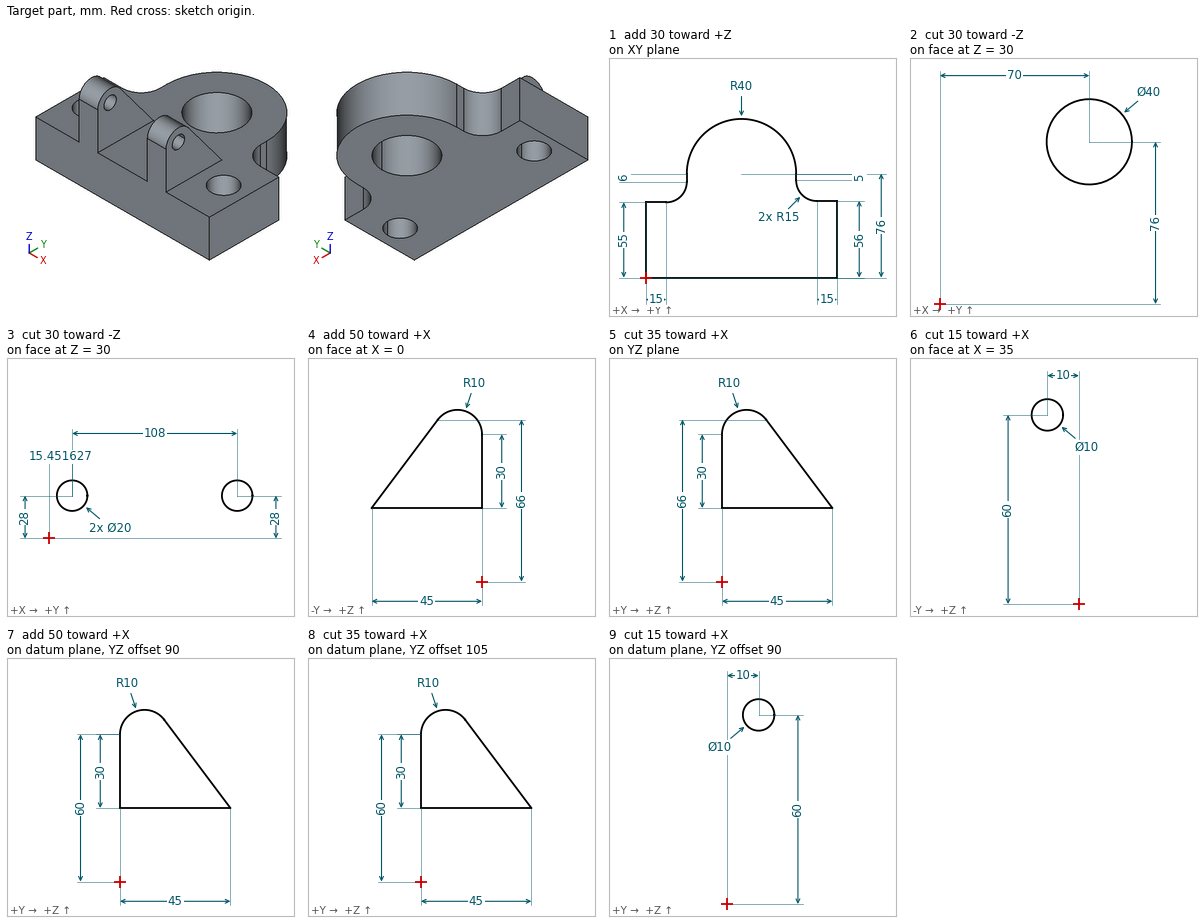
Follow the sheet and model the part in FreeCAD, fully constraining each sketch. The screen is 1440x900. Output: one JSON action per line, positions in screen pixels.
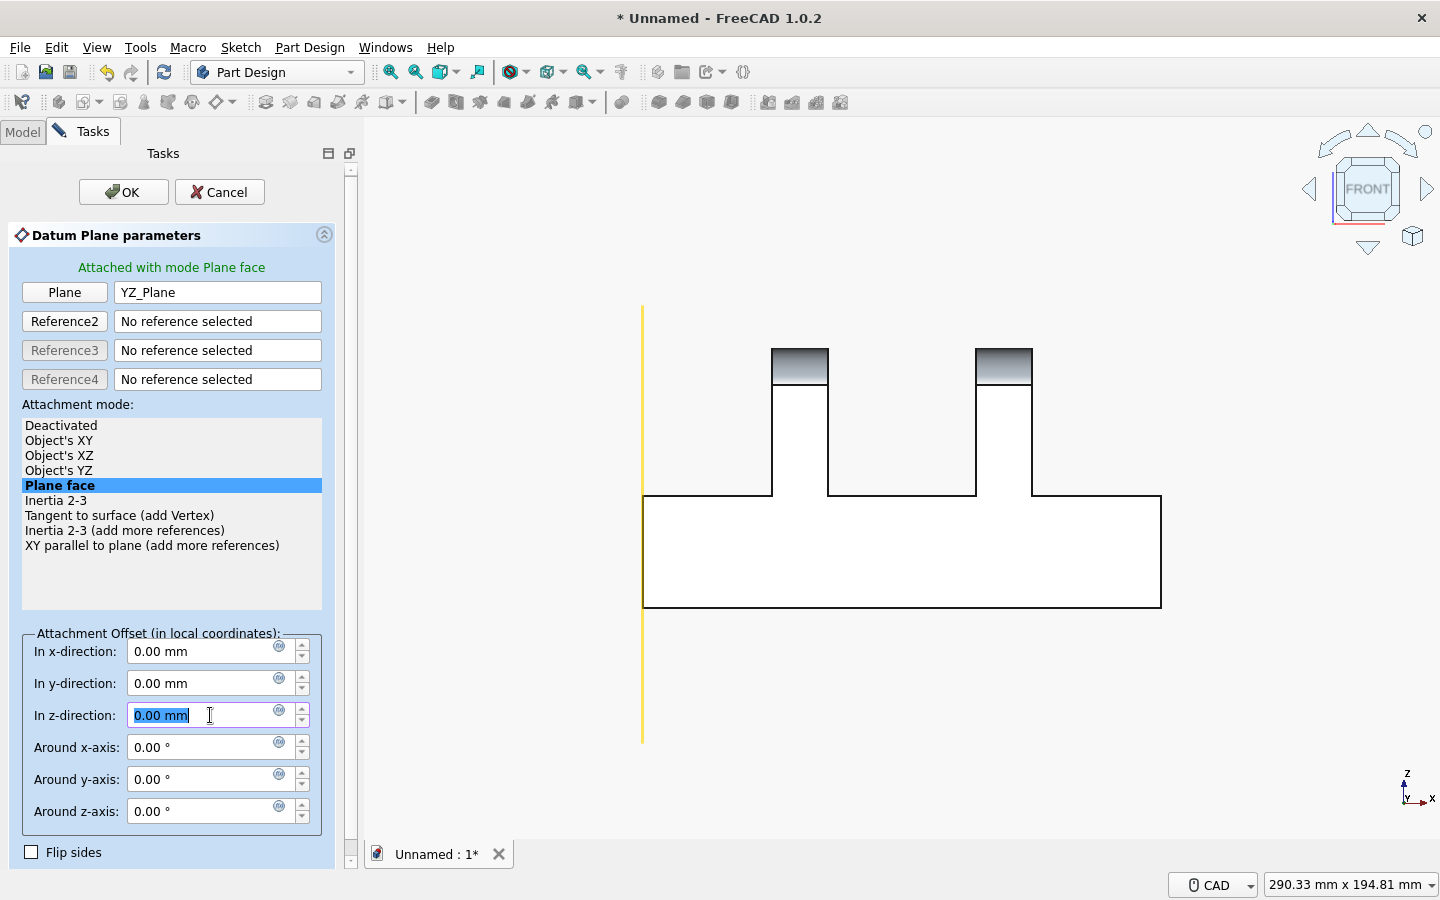
{"action": "type", "text": "90"}
{"action": "key", "text": "Tab"}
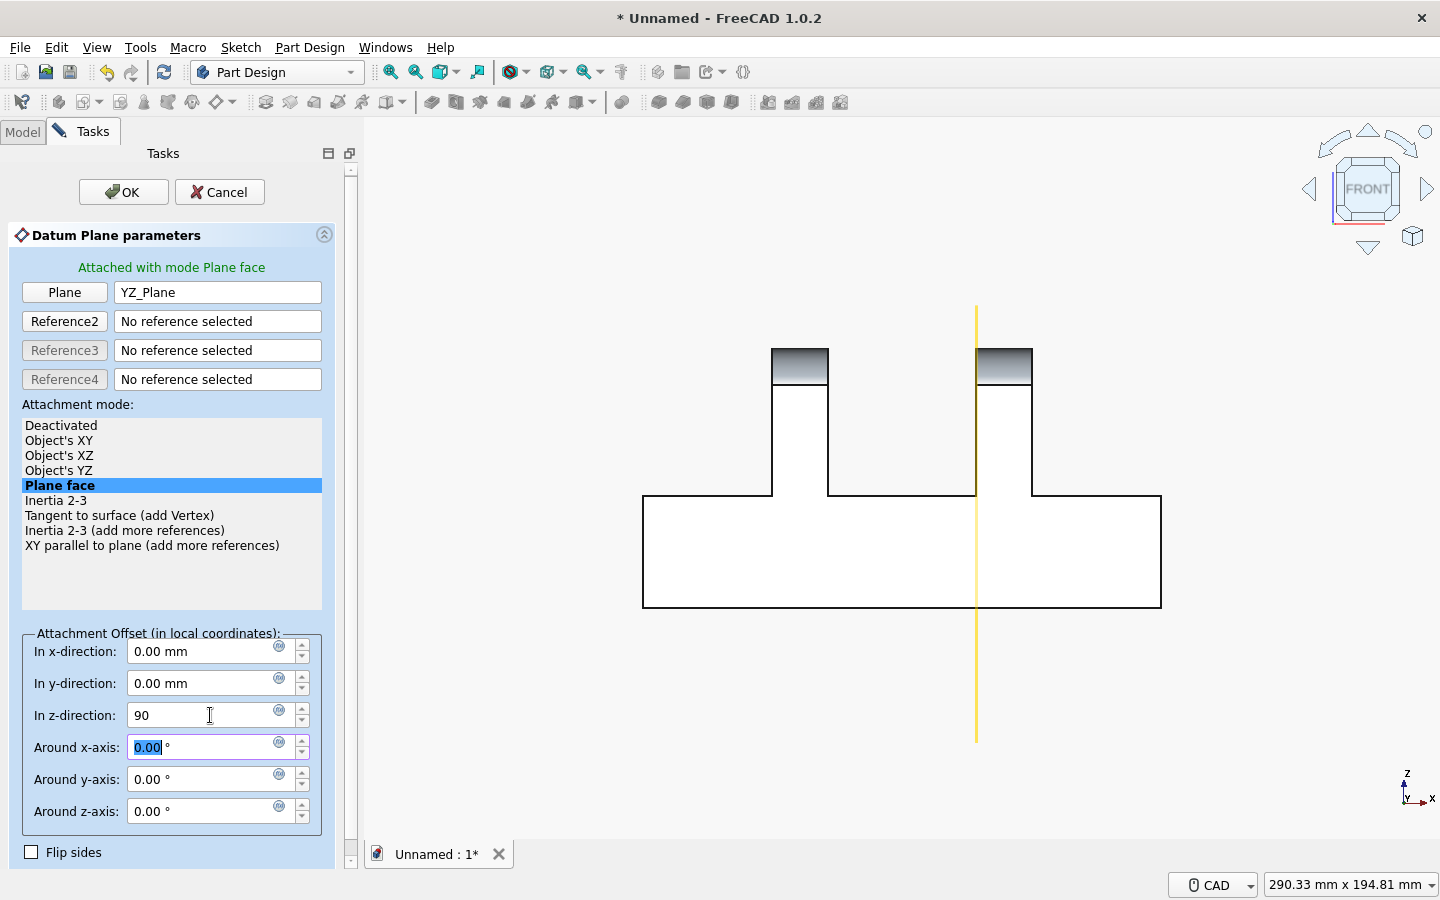
{"action": "left_click", "coordinate": [124, 192]}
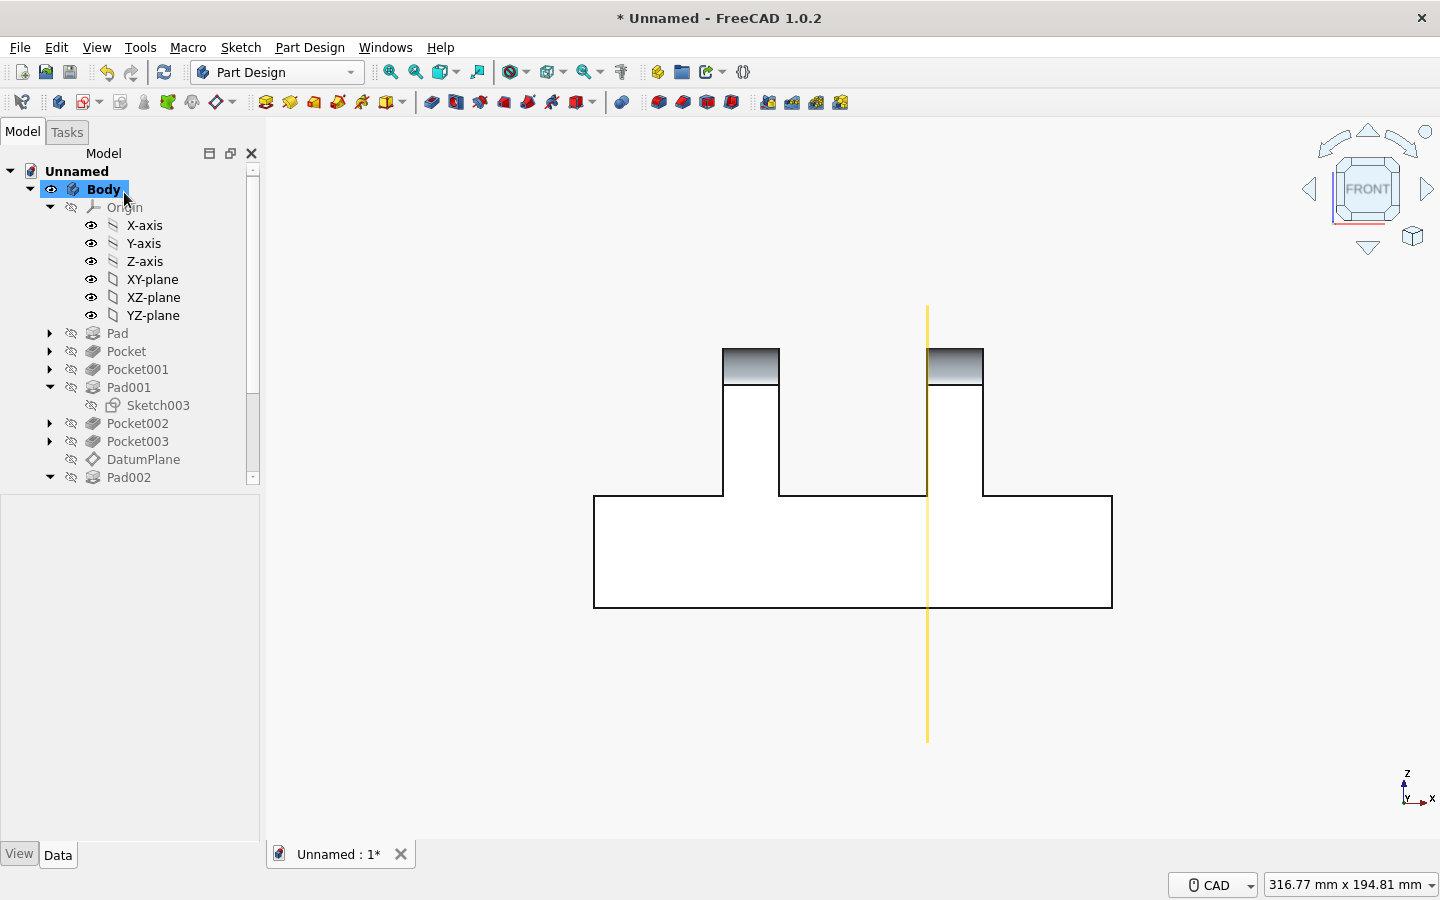
{"action": "scroll", "coordinate": [100, 329], "scroll_direction": "down", "scroll_amount": 3}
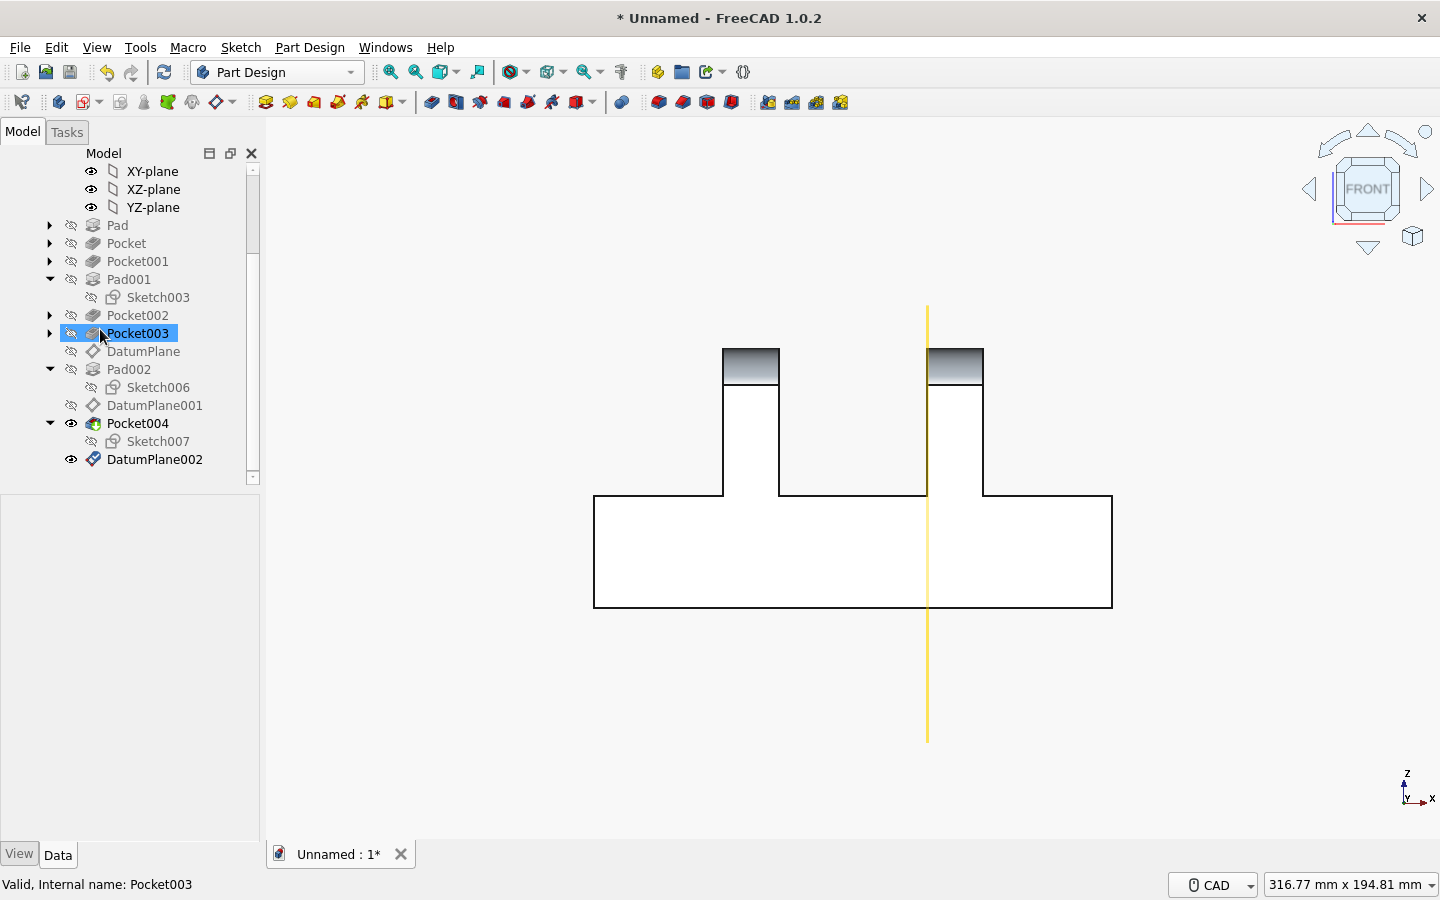
{"action": "left_click", "coordinate": [116, 459]}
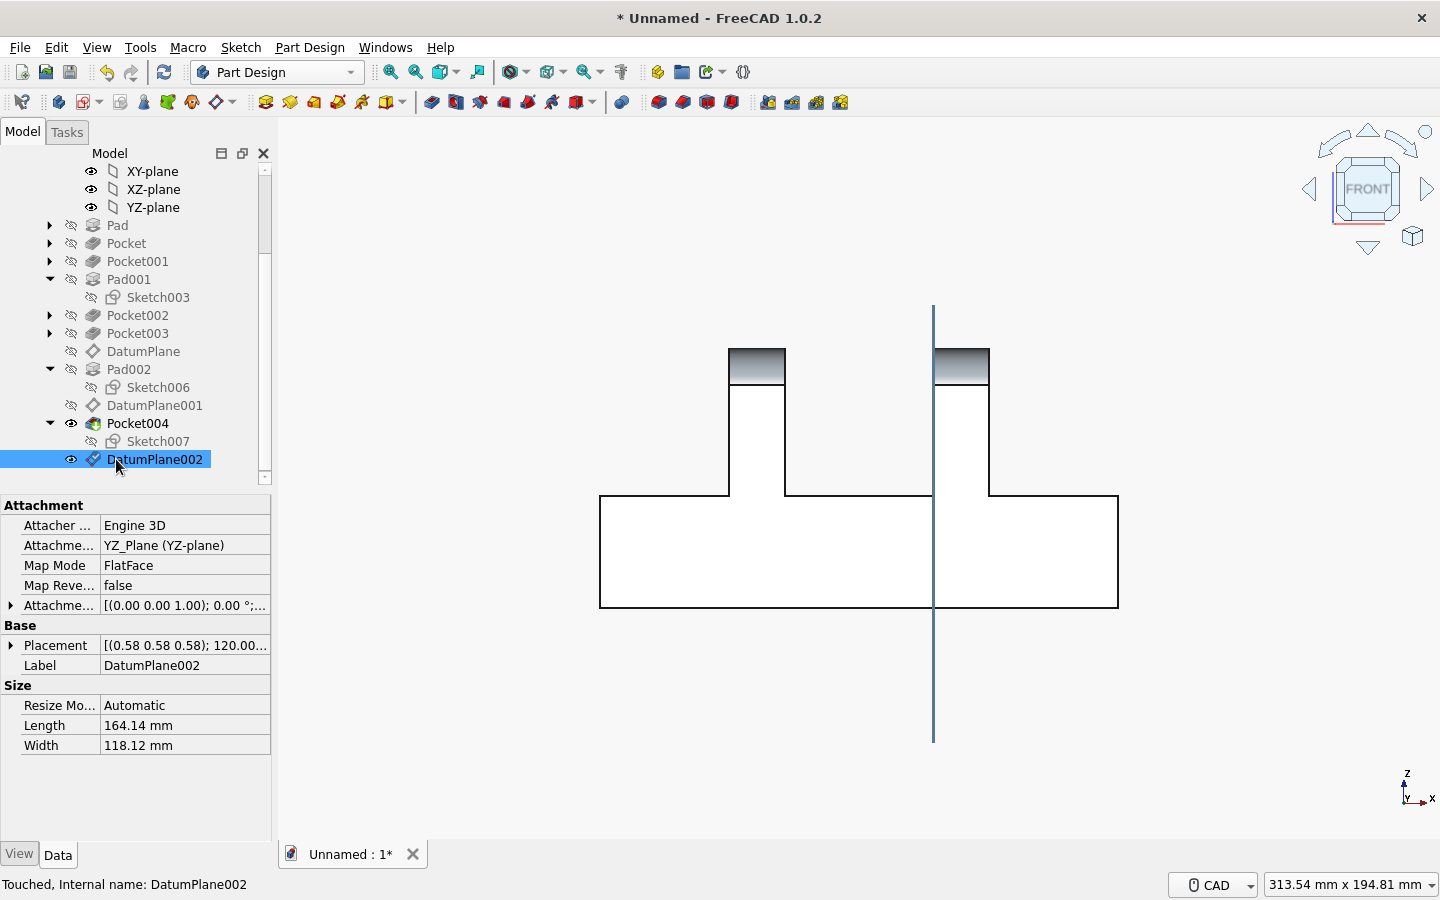
{"action": "left_click", "coordinate": [84, 102]}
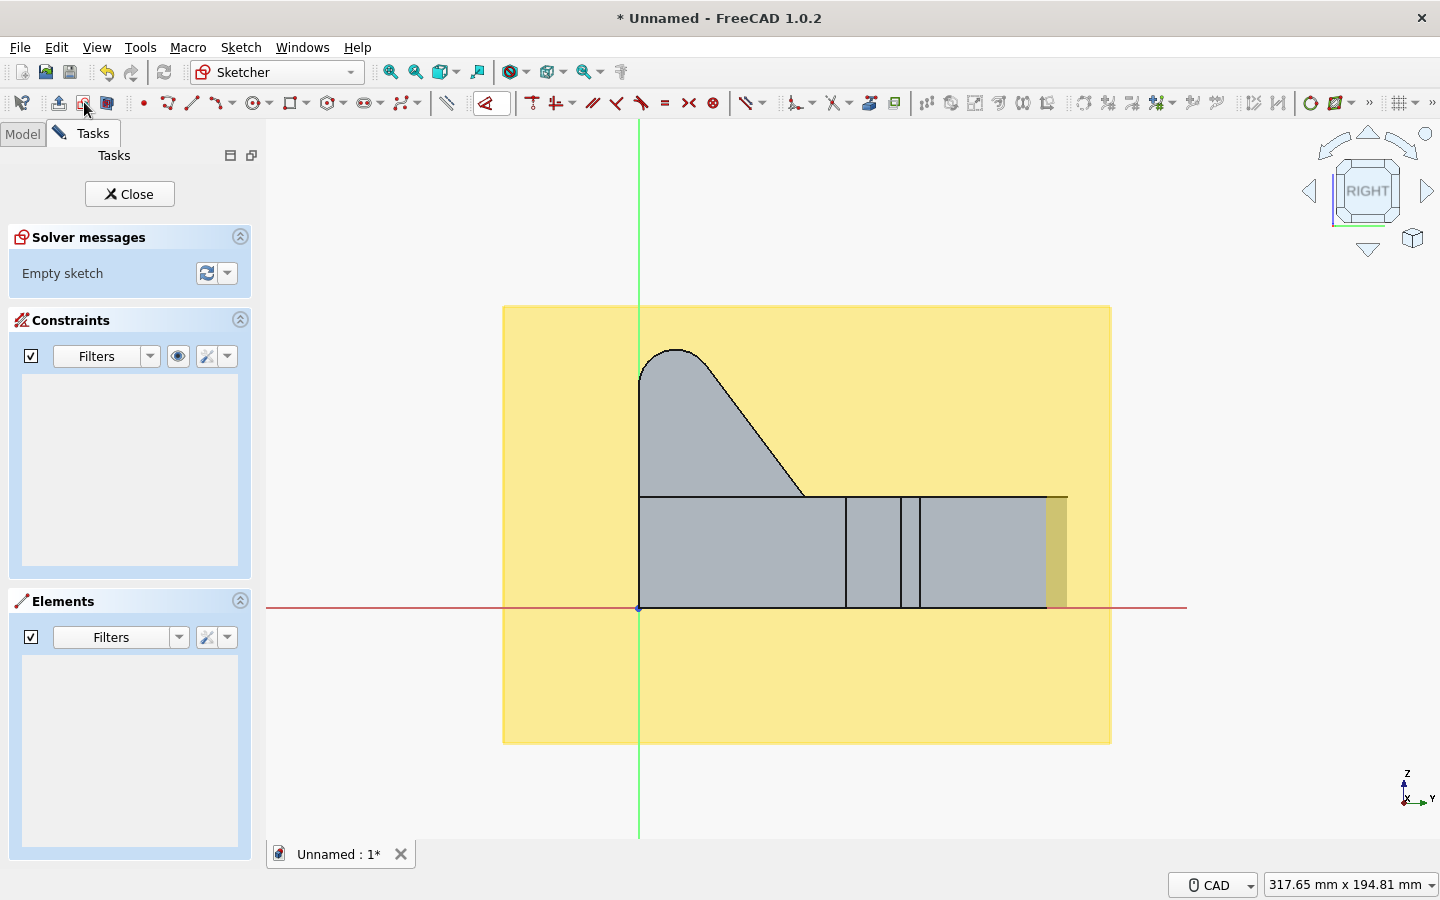
{"action": "key", "text": "q s"}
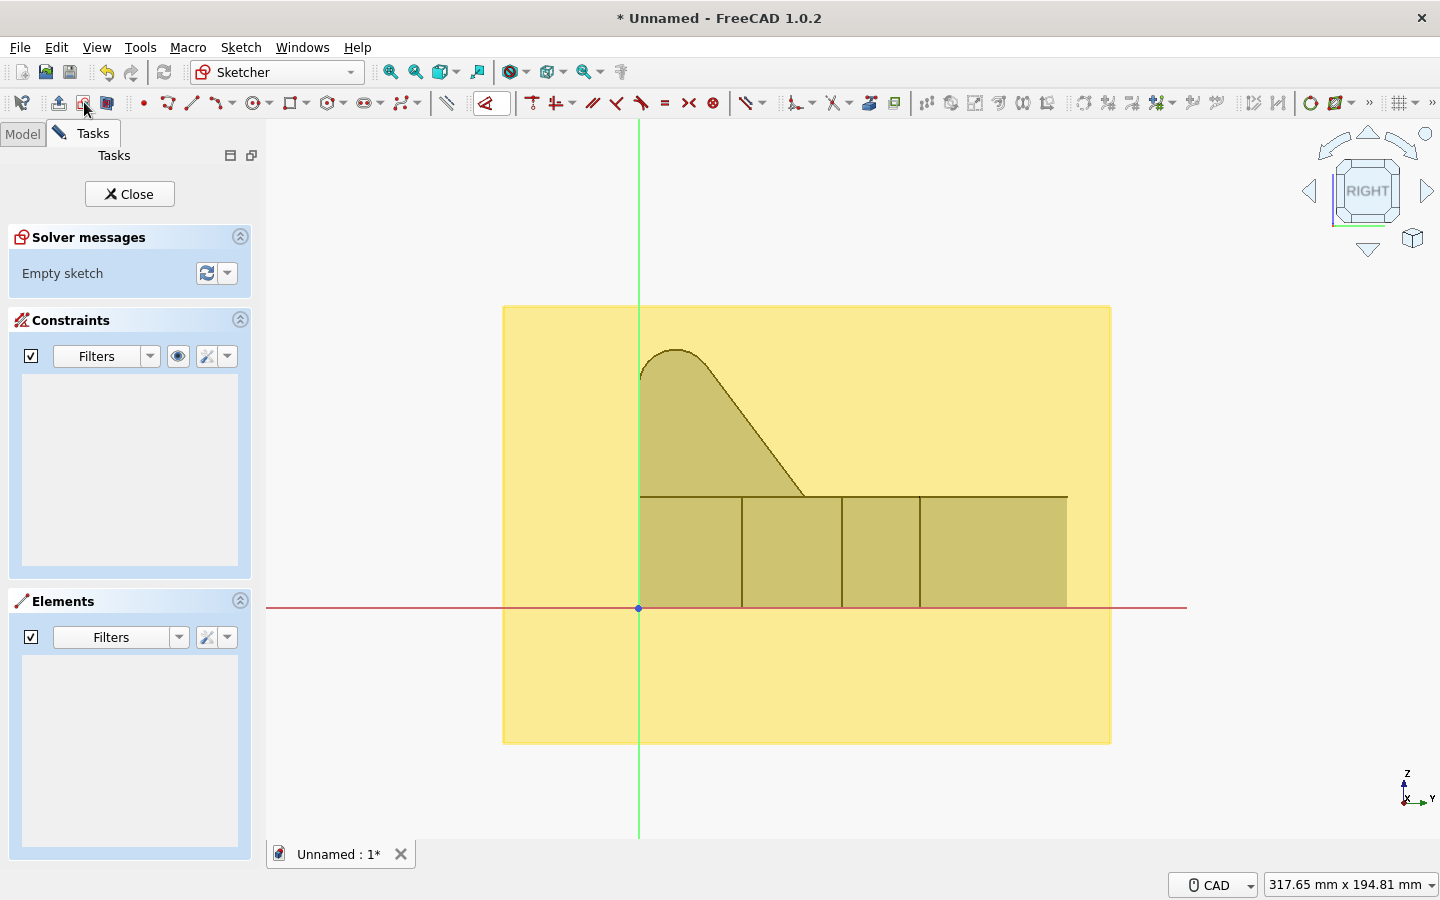
{"action": "scroll", "coordinate": [667, 379], "scroll_direction": "up", "scroll_amount": 13}